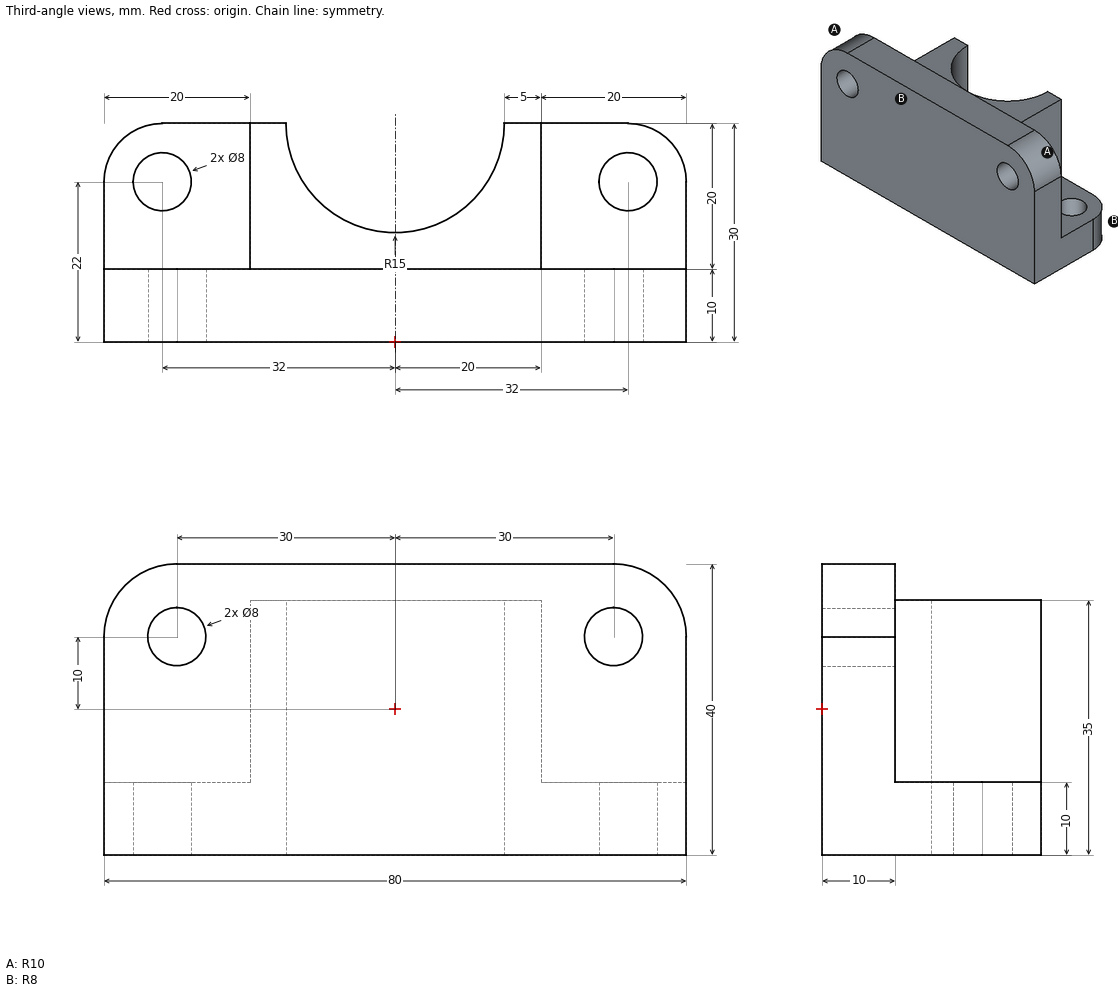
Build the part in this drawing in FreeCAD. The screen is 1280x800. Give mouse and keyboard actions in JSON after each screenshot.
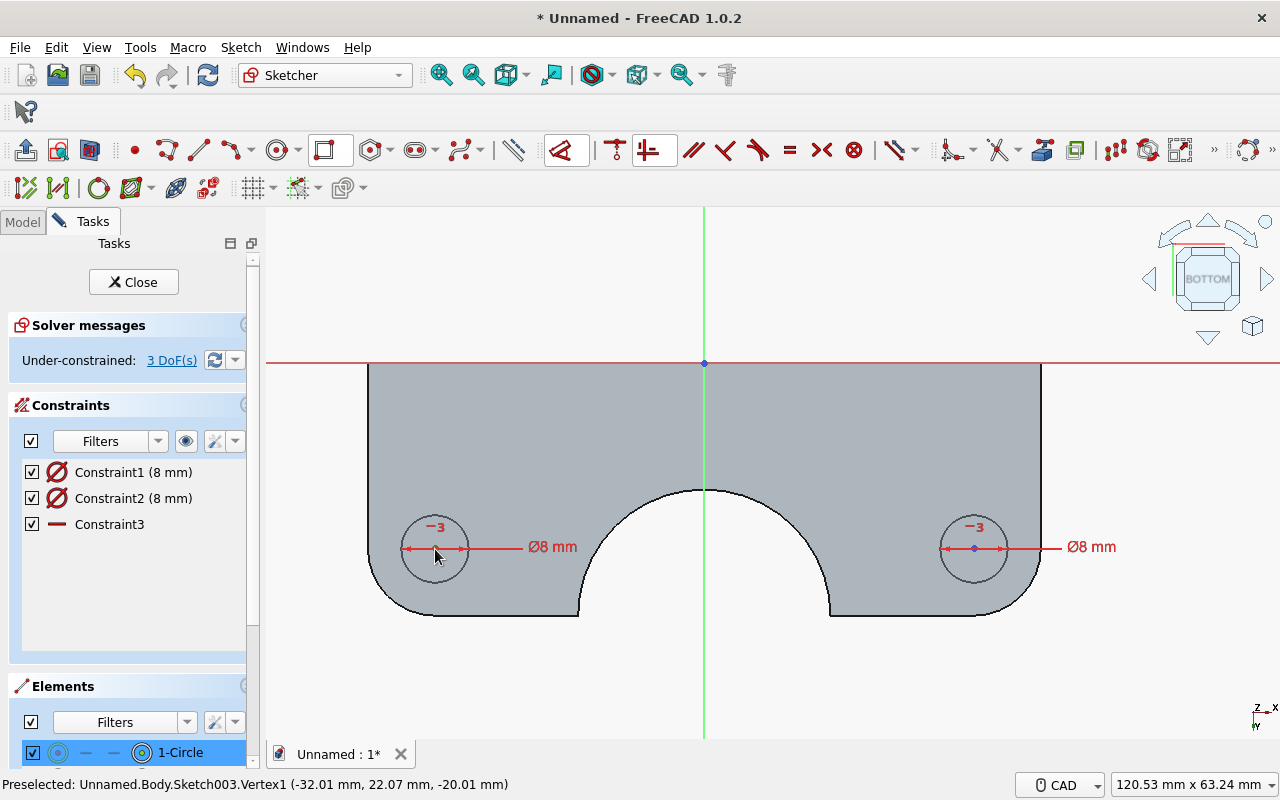
{"action": "key", "text": "l"}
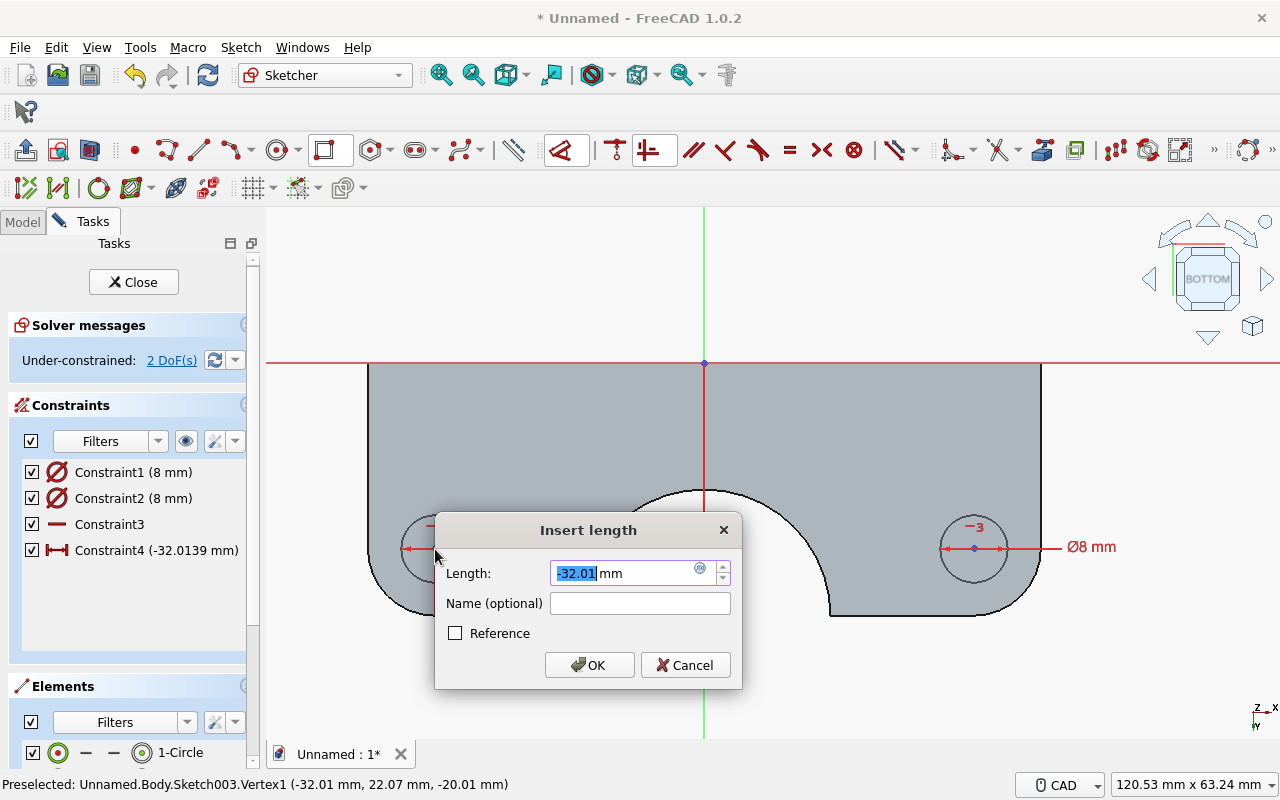
{"action": "type", "text": "-32"}
{"action": "key", "text": "Return"}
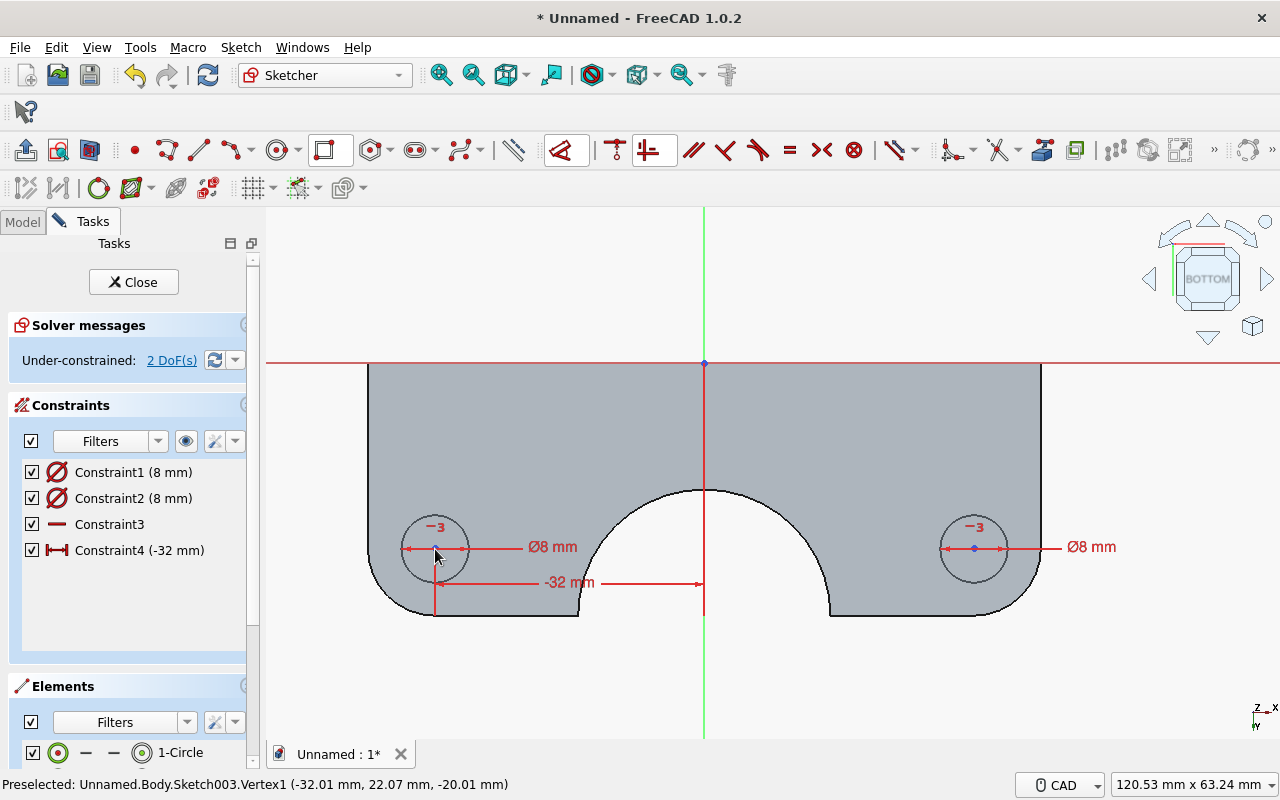
{"action": "left_click", "coordinate": [435, 549]}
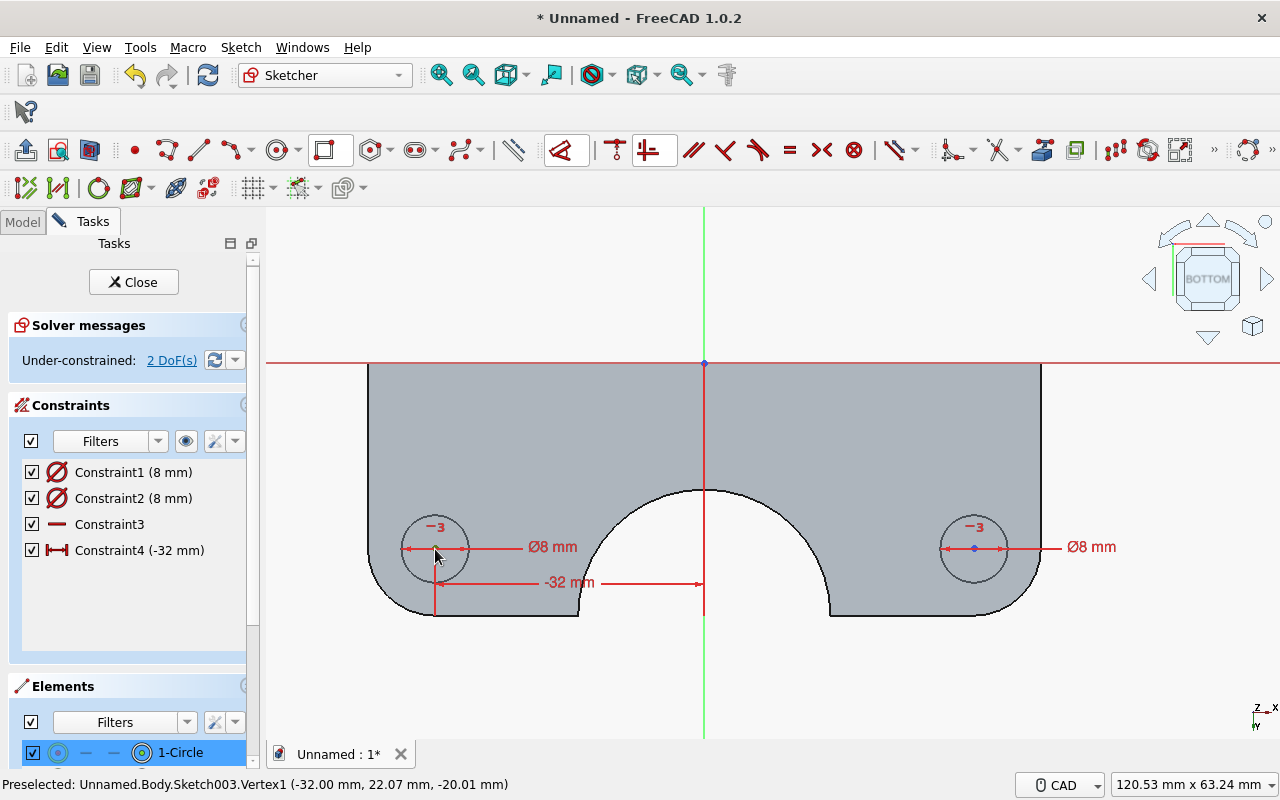
{"action": "left_click", "coordinate": [584, 150]}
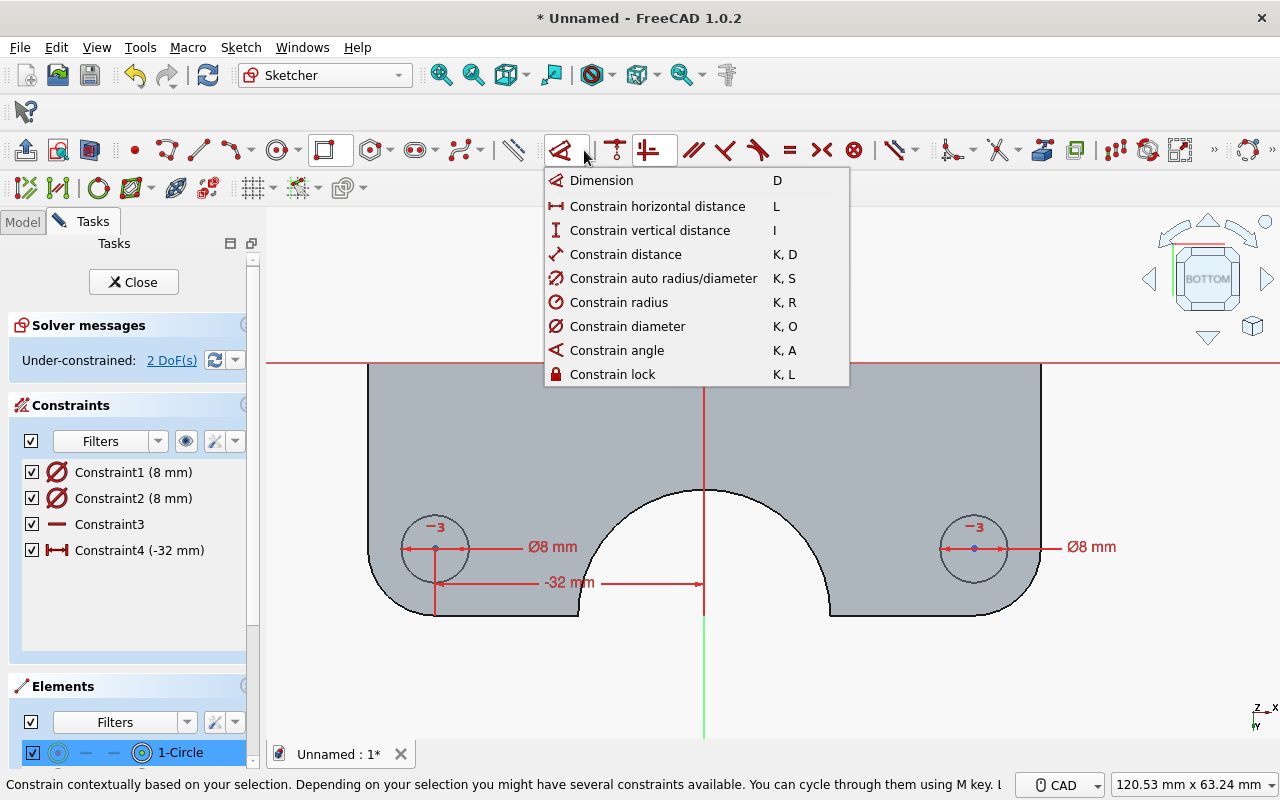
{"action": "left_click", "coordinate": [697, 230]}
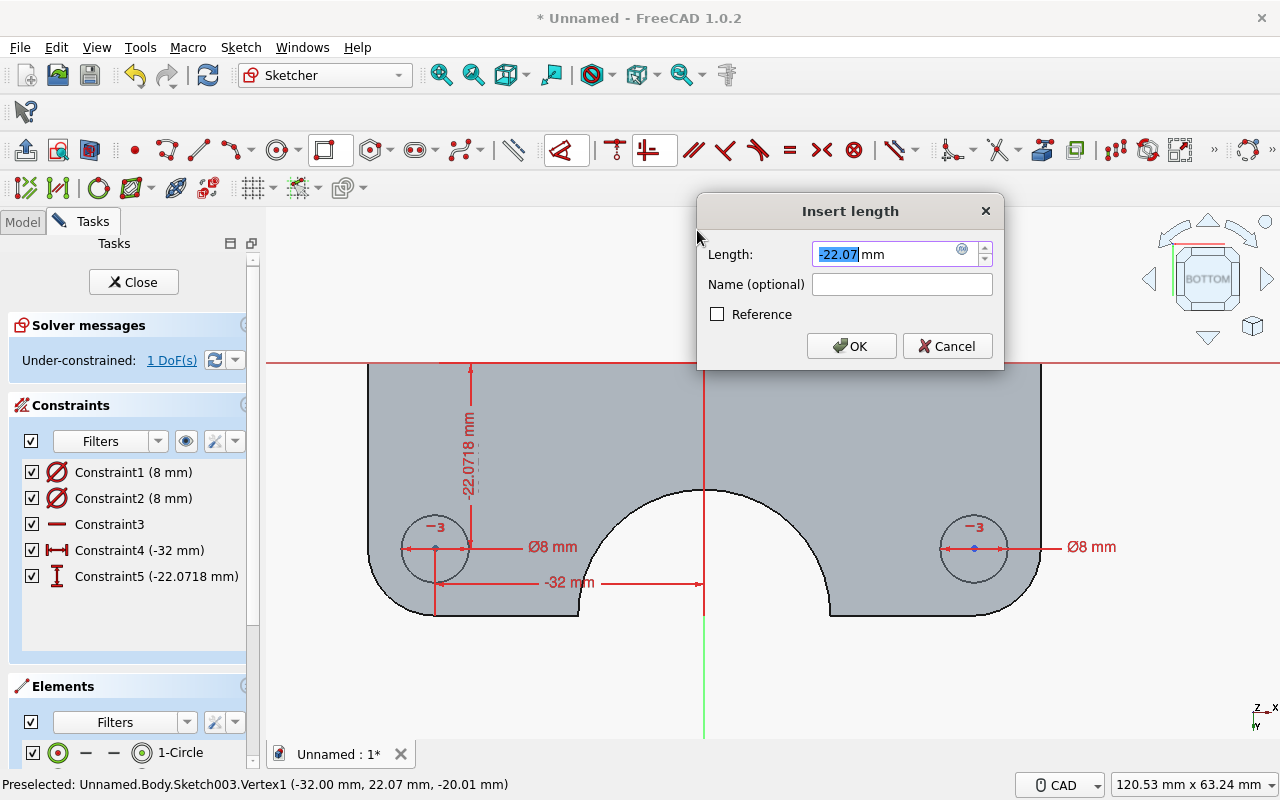
{"action": "type", "text": "-22"}
{"action": "key", "text": "Return"}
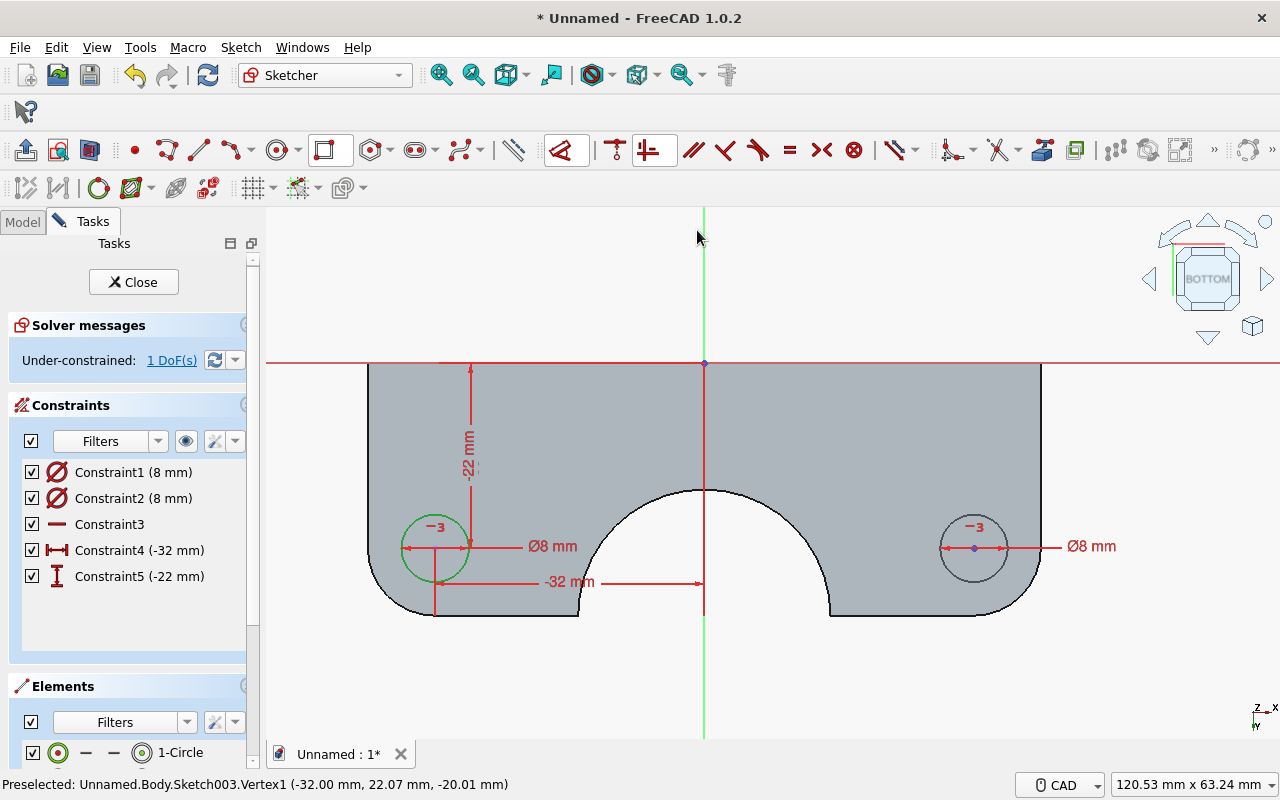
{"action": "left_click", "coordinate": [974, 548]}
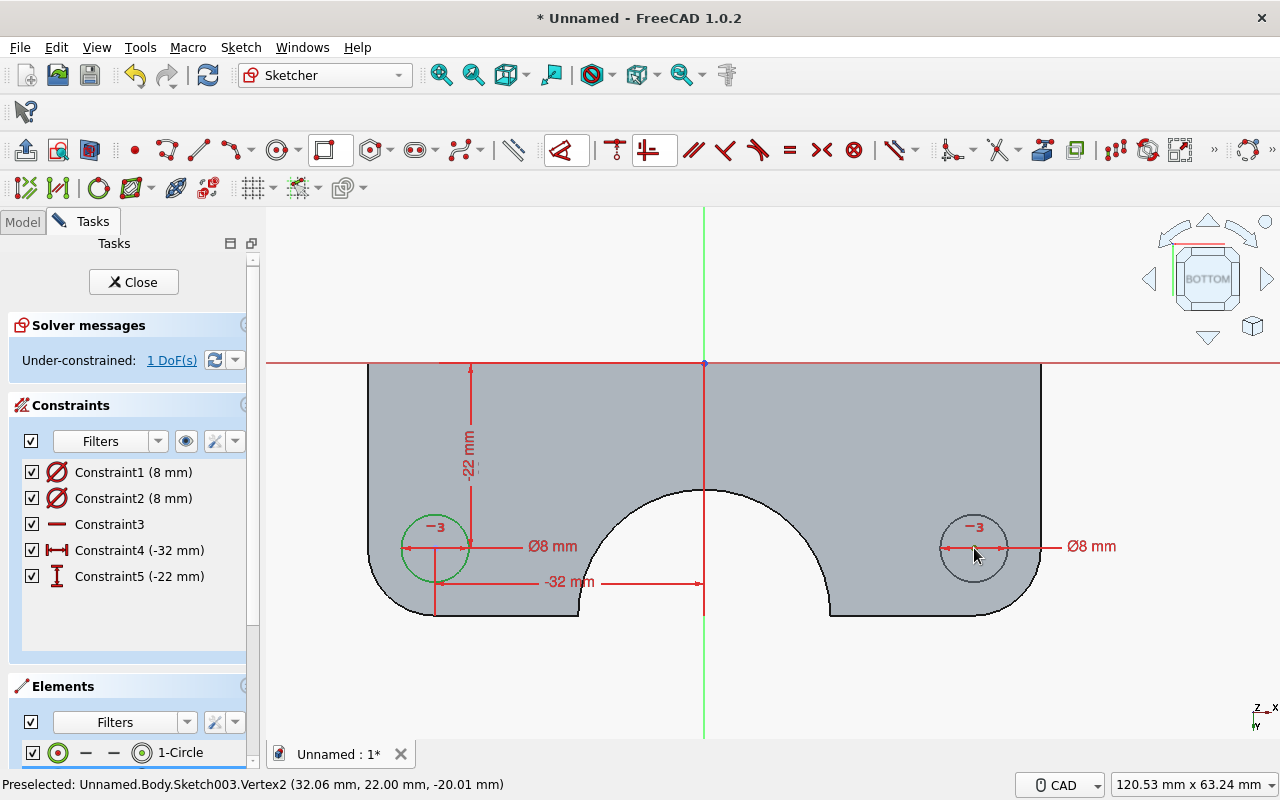
{"action": "key", "text": "l"}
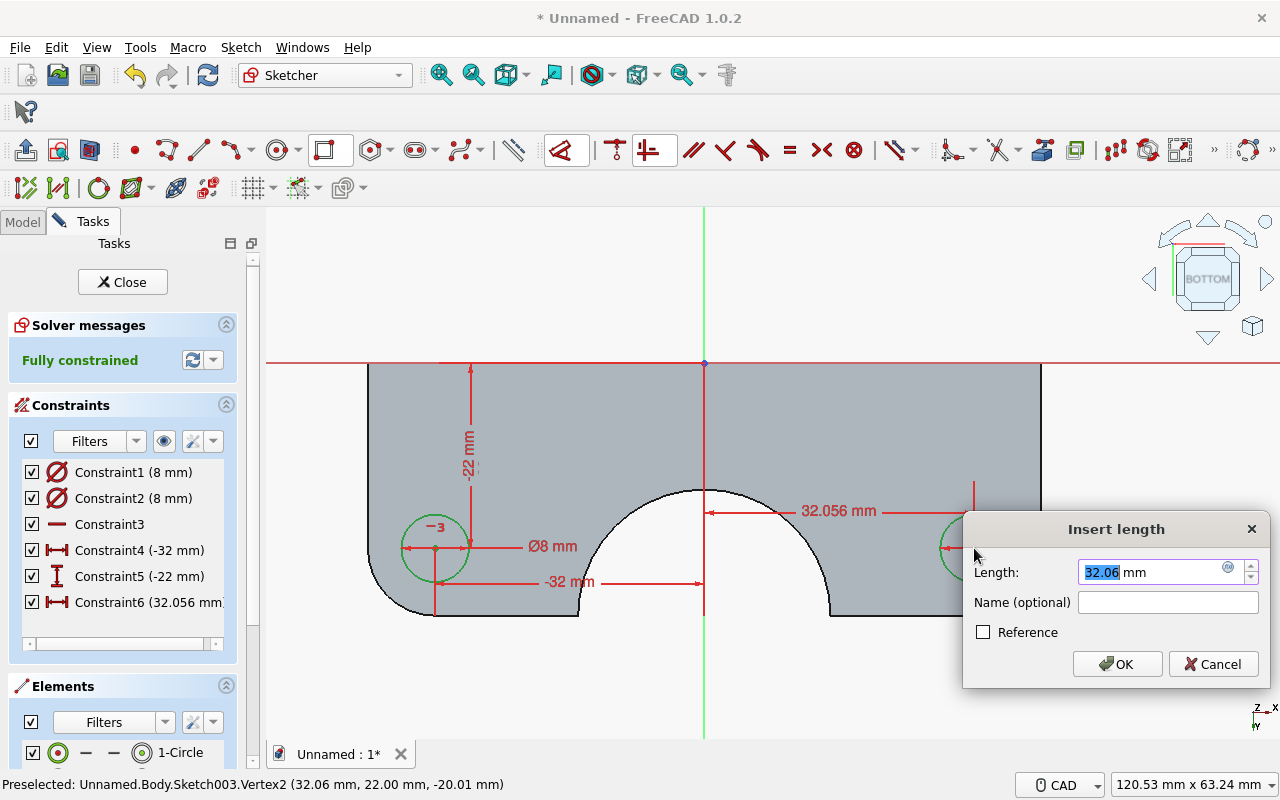
{"action": "type", "text": "32"}
{"action": "key", "text": "Return"}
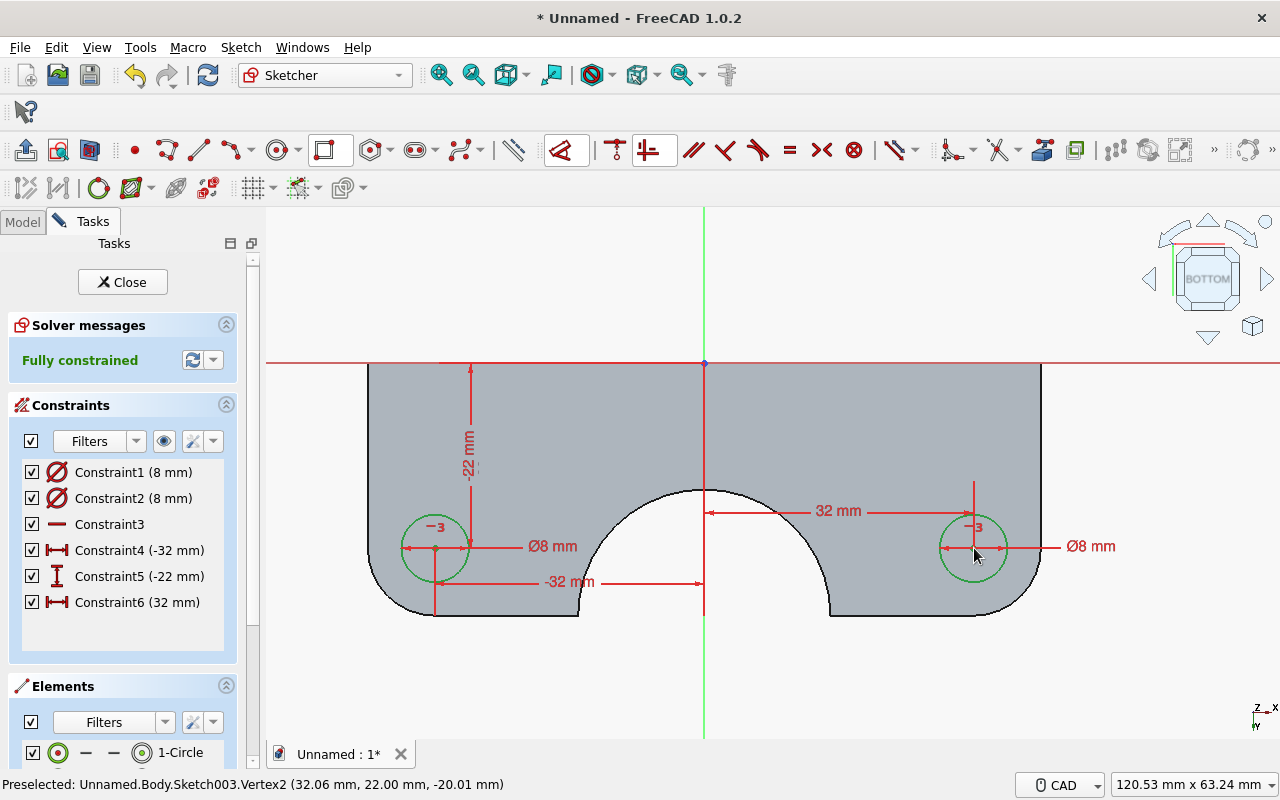
{"action": "left_click", "coordinate": [123, 282]}